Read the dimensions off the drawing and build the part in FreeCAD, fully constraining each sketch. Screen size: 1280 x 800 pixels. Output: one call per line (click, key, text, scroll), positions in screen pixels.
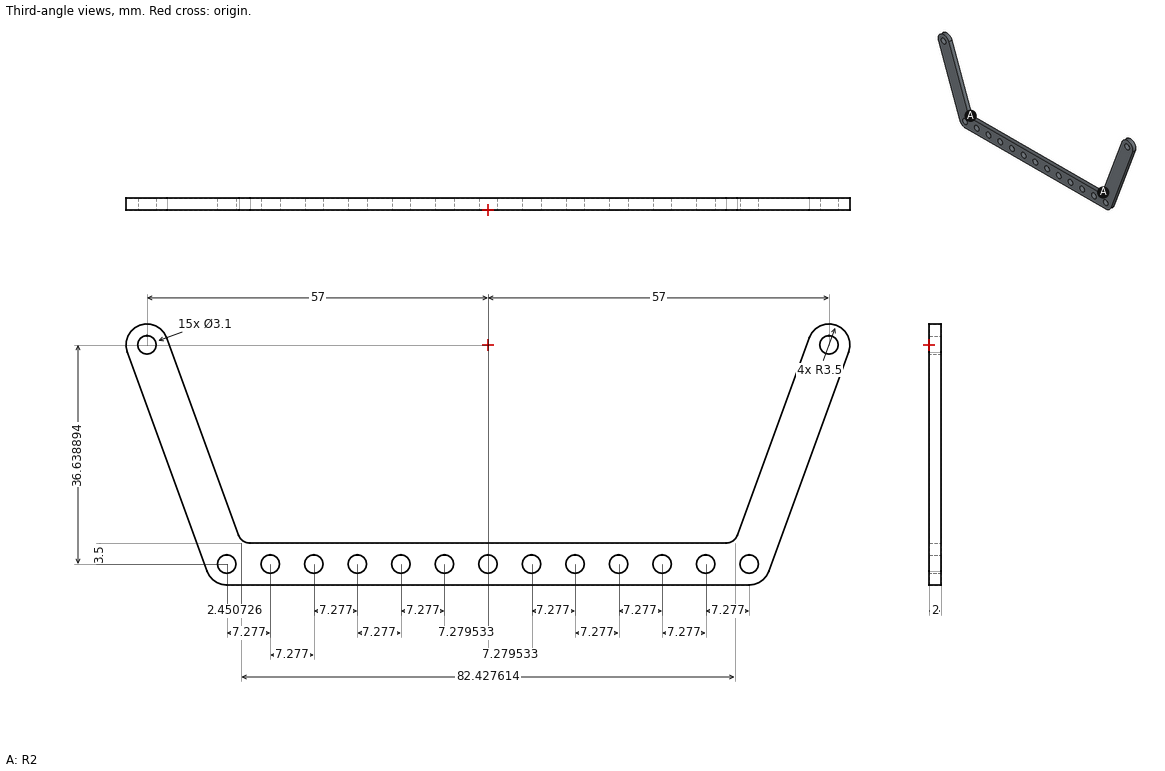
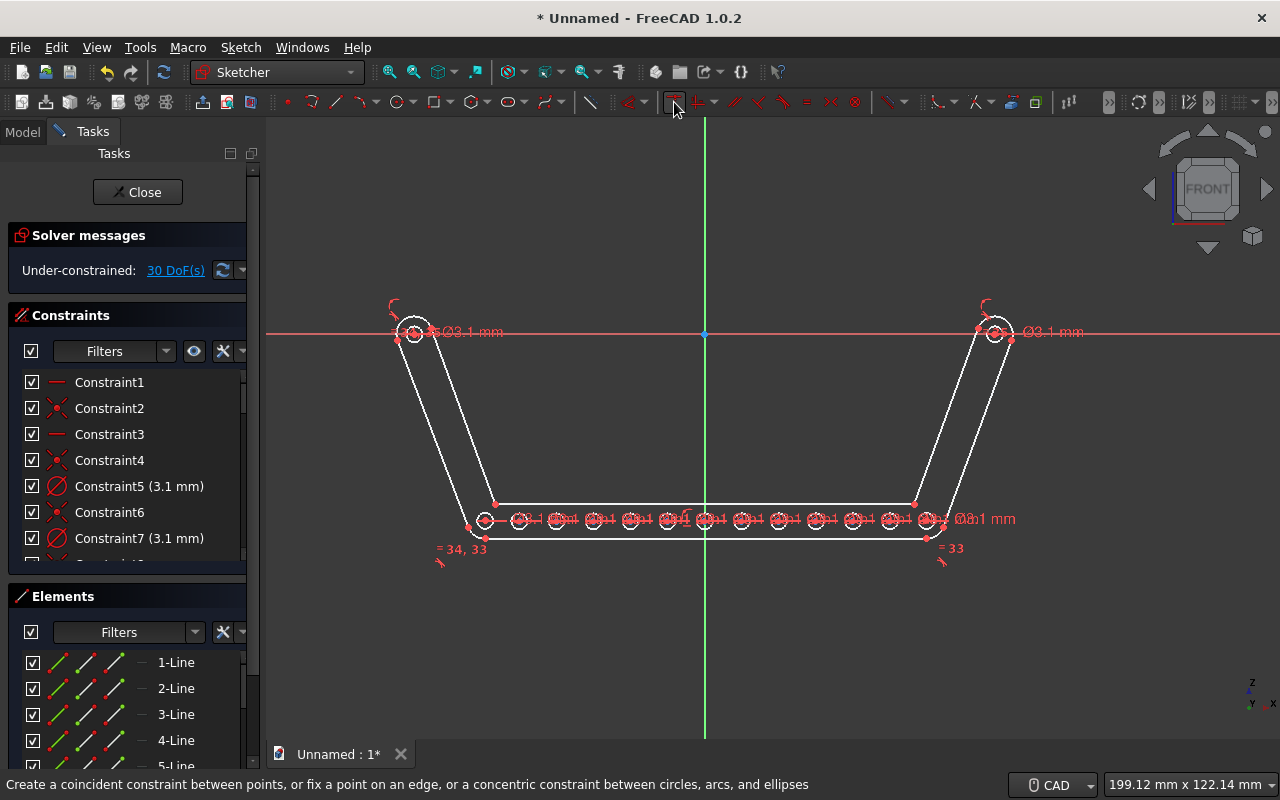
key(d)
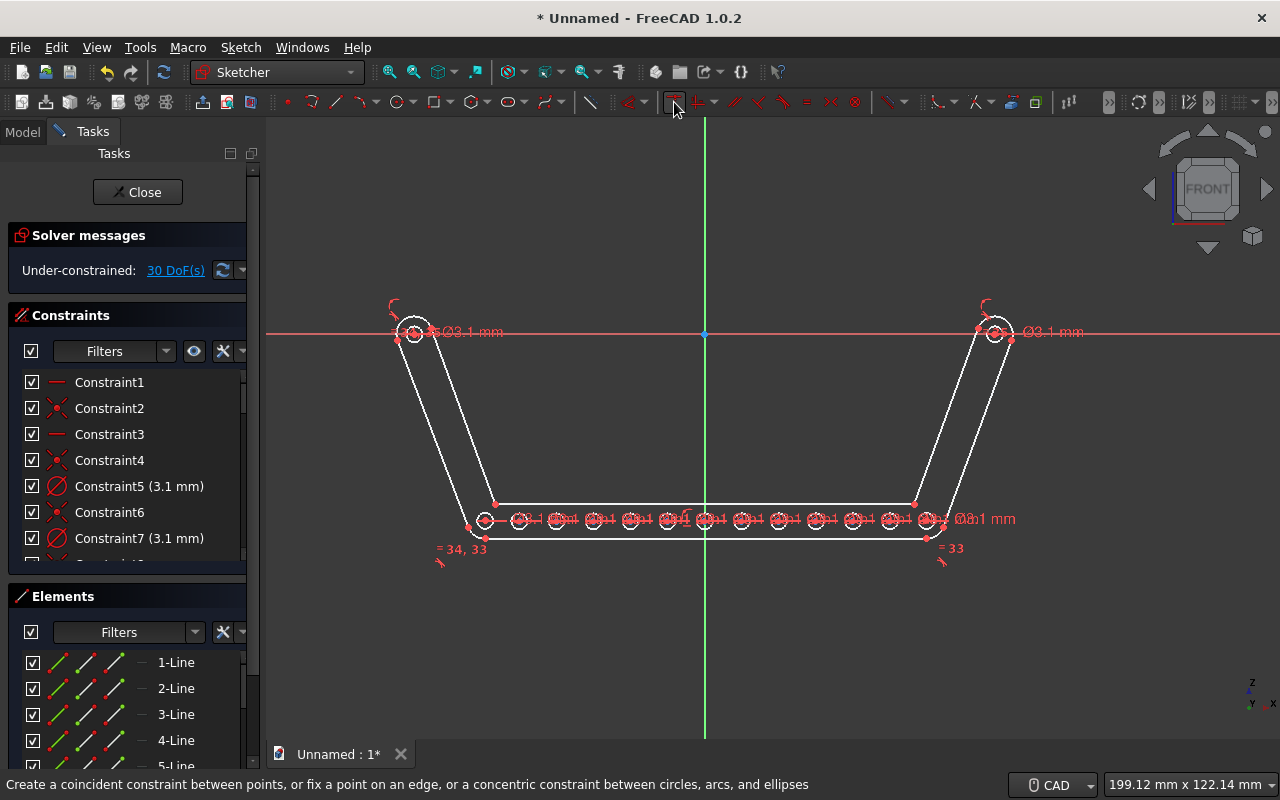
scroll(937, 536, up, 5)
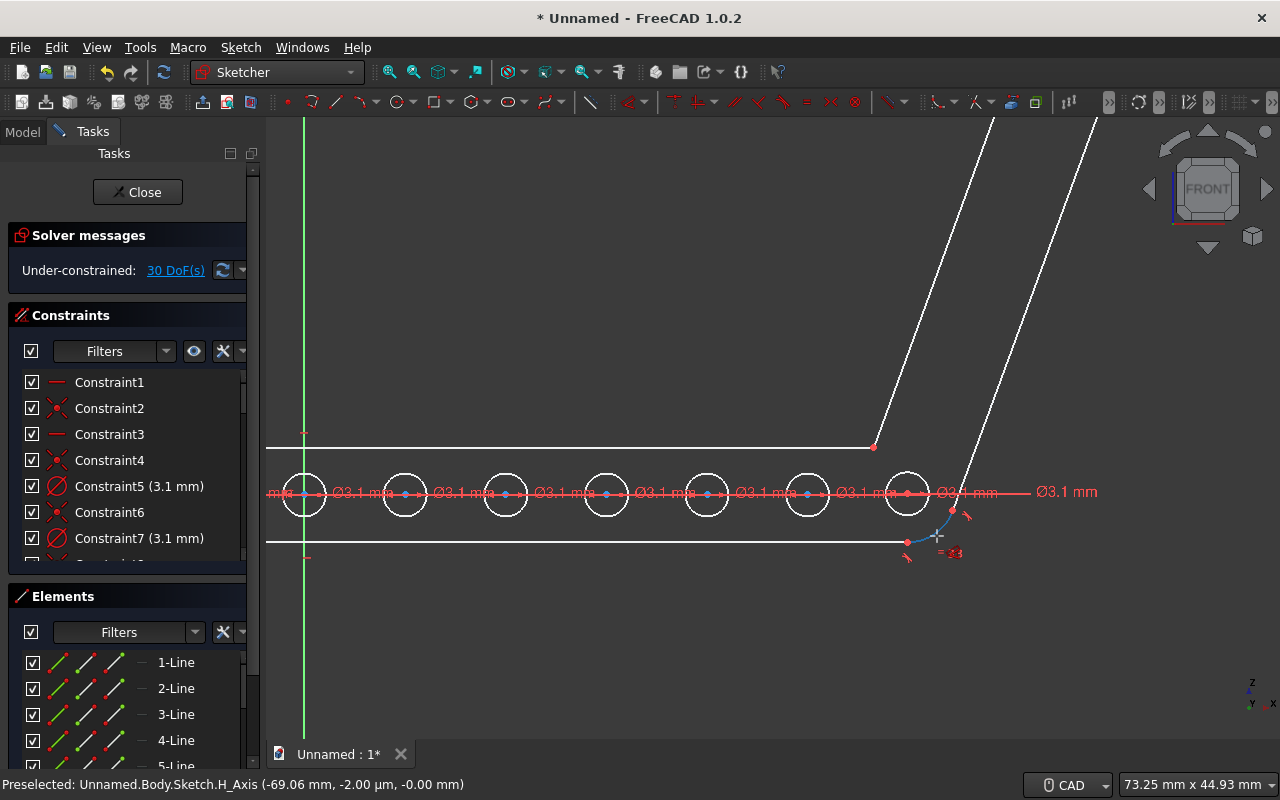
click(935, 534)
click(953, 560)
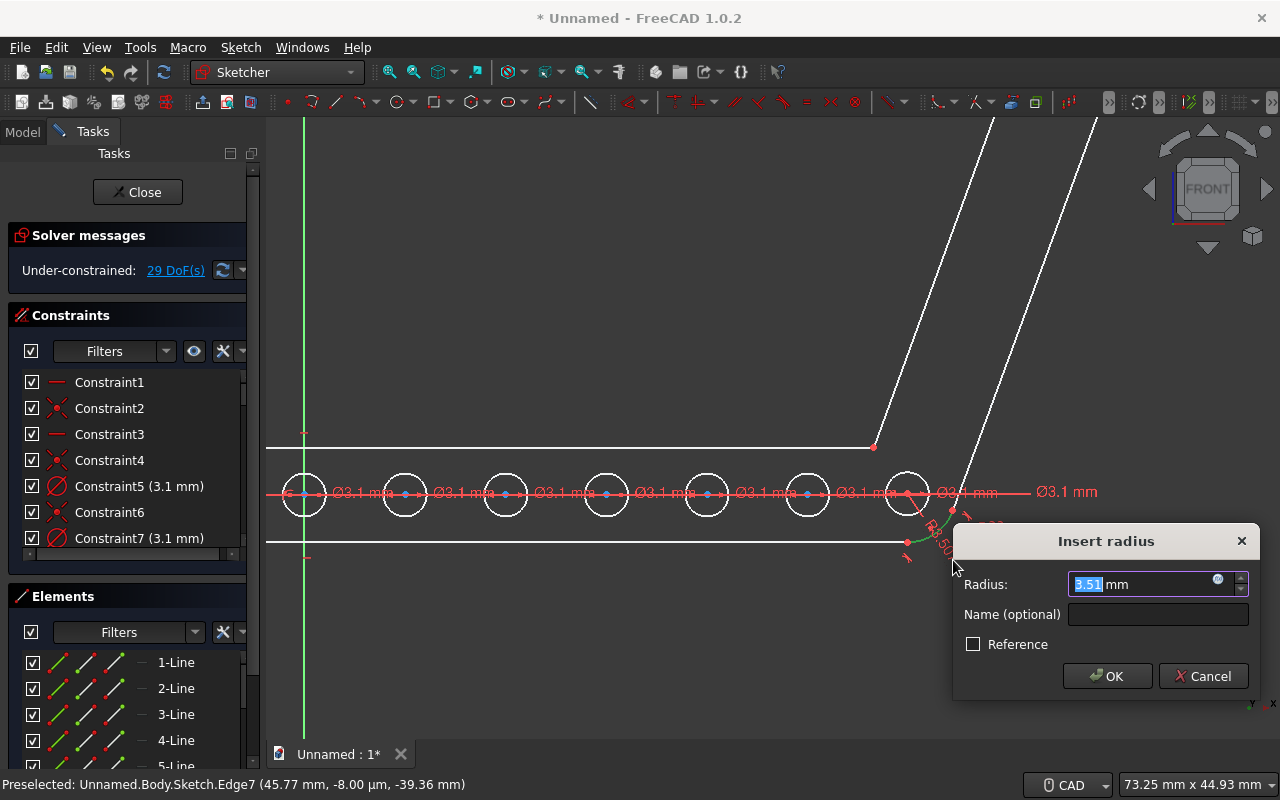
text(3.5)
key(Return)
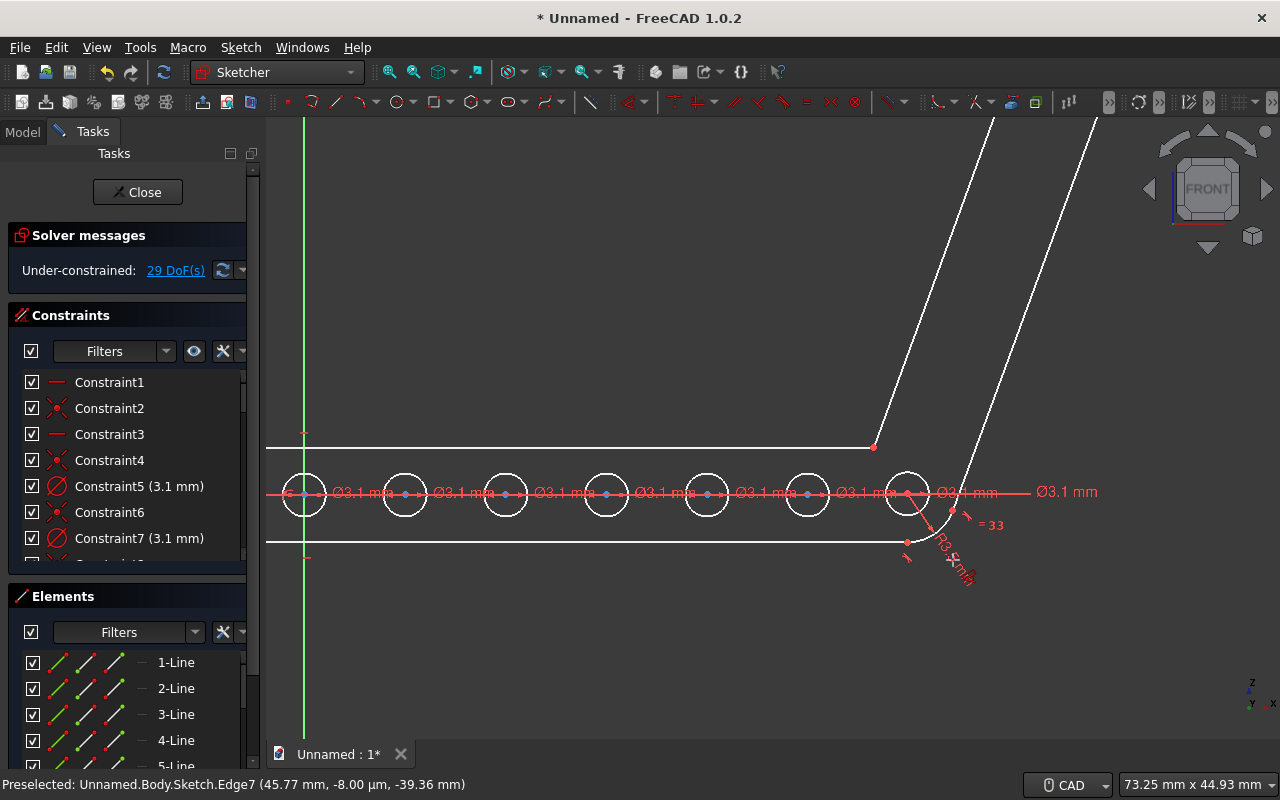
scroll(937, 536, down, 5)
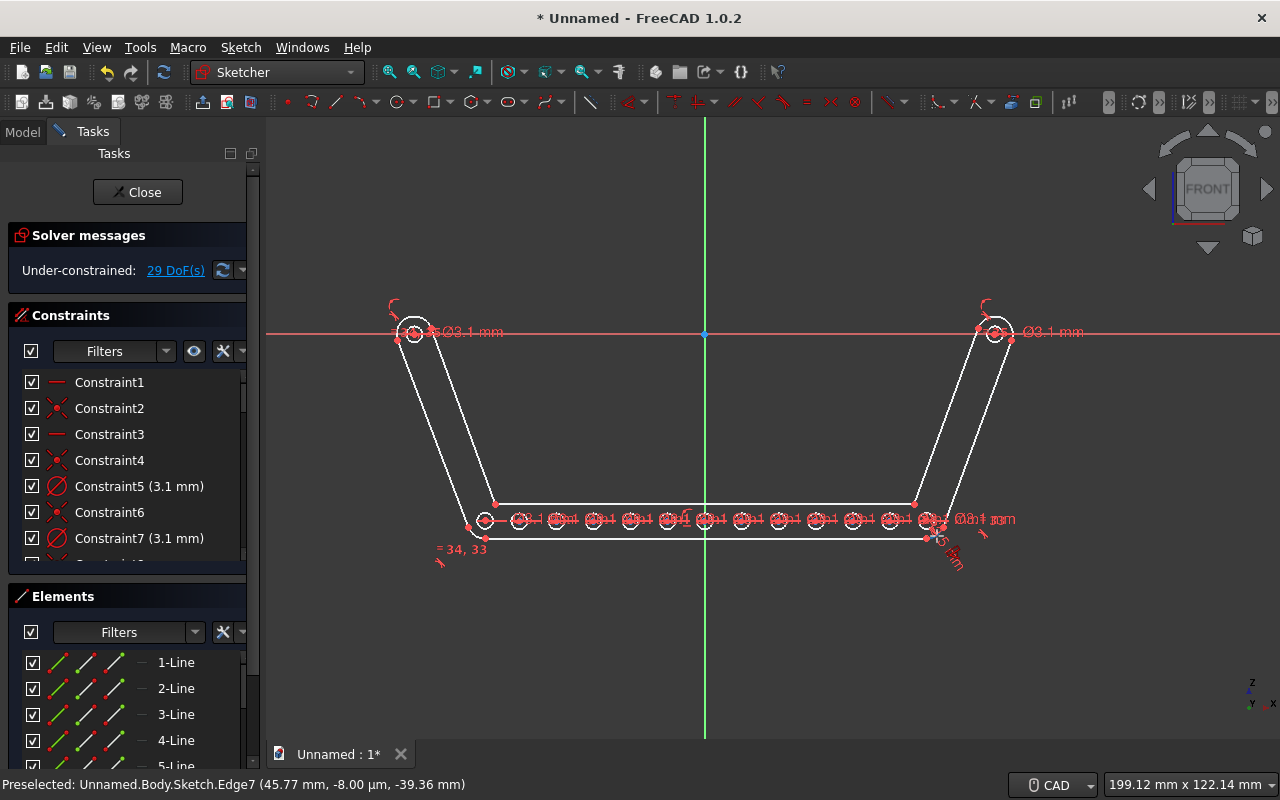
click(414, 334)
click(560, 300)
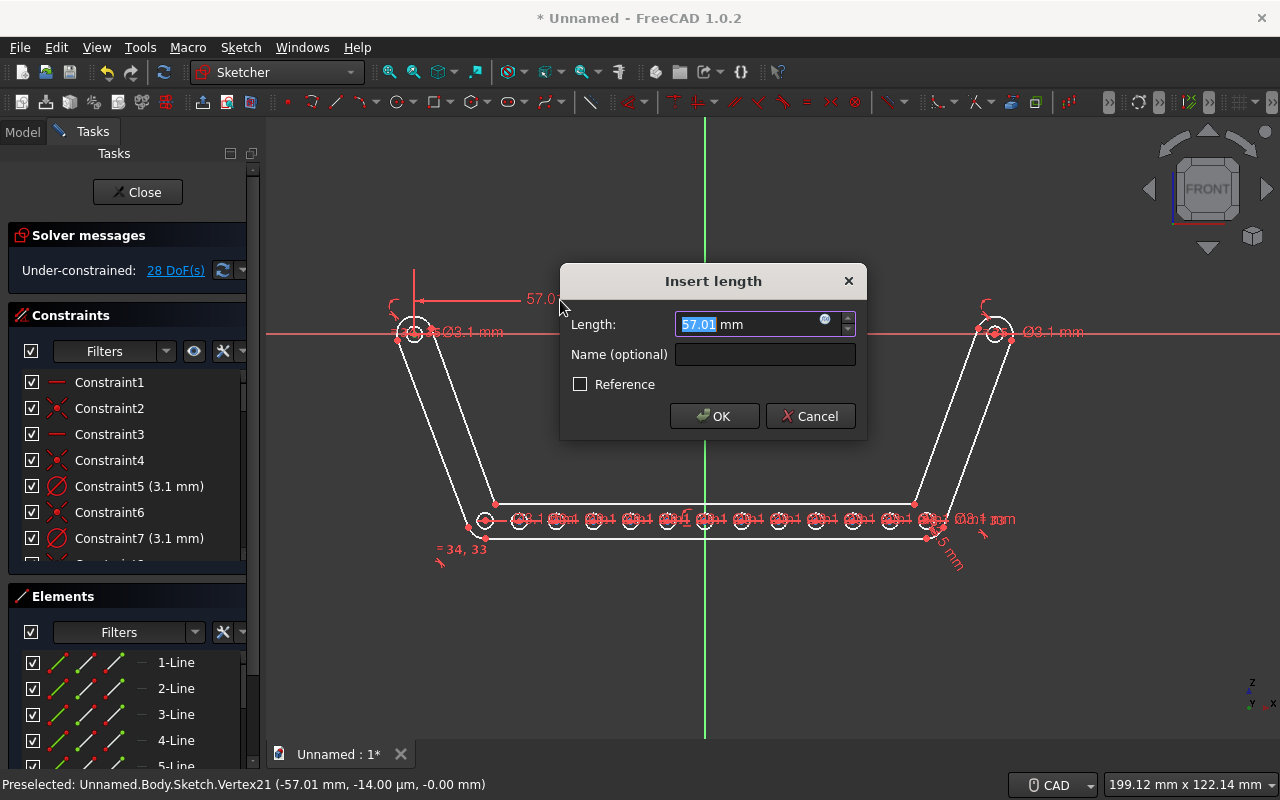
text(57)
key(Return)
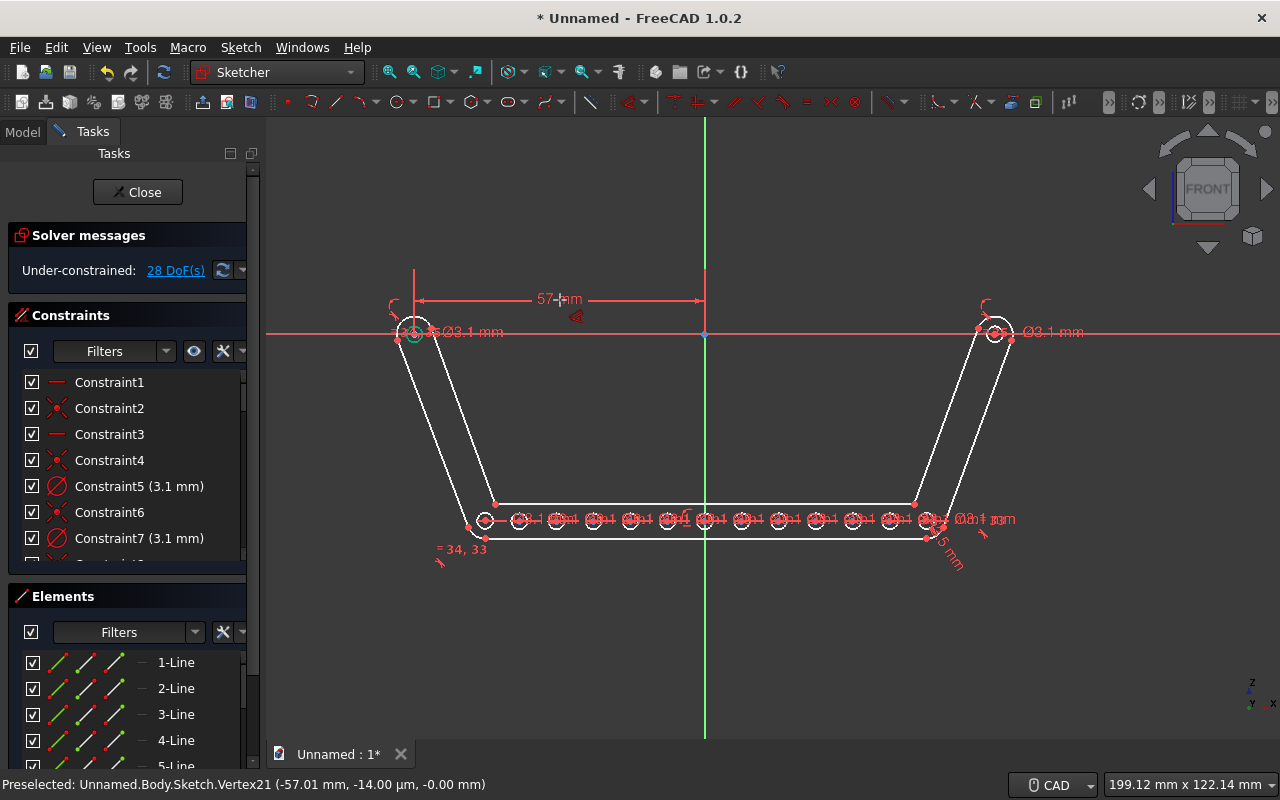
click(995, 334)
click(850, 300)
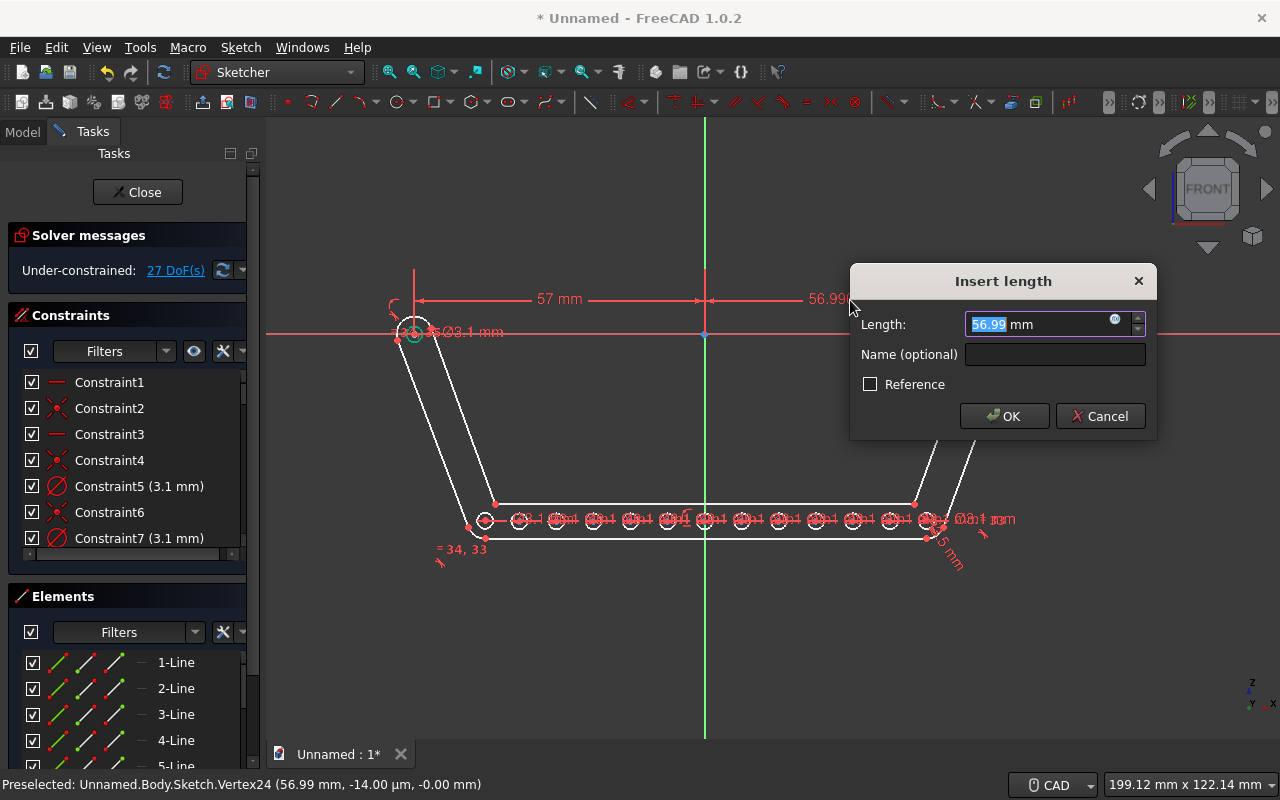
text(57)
key(Return)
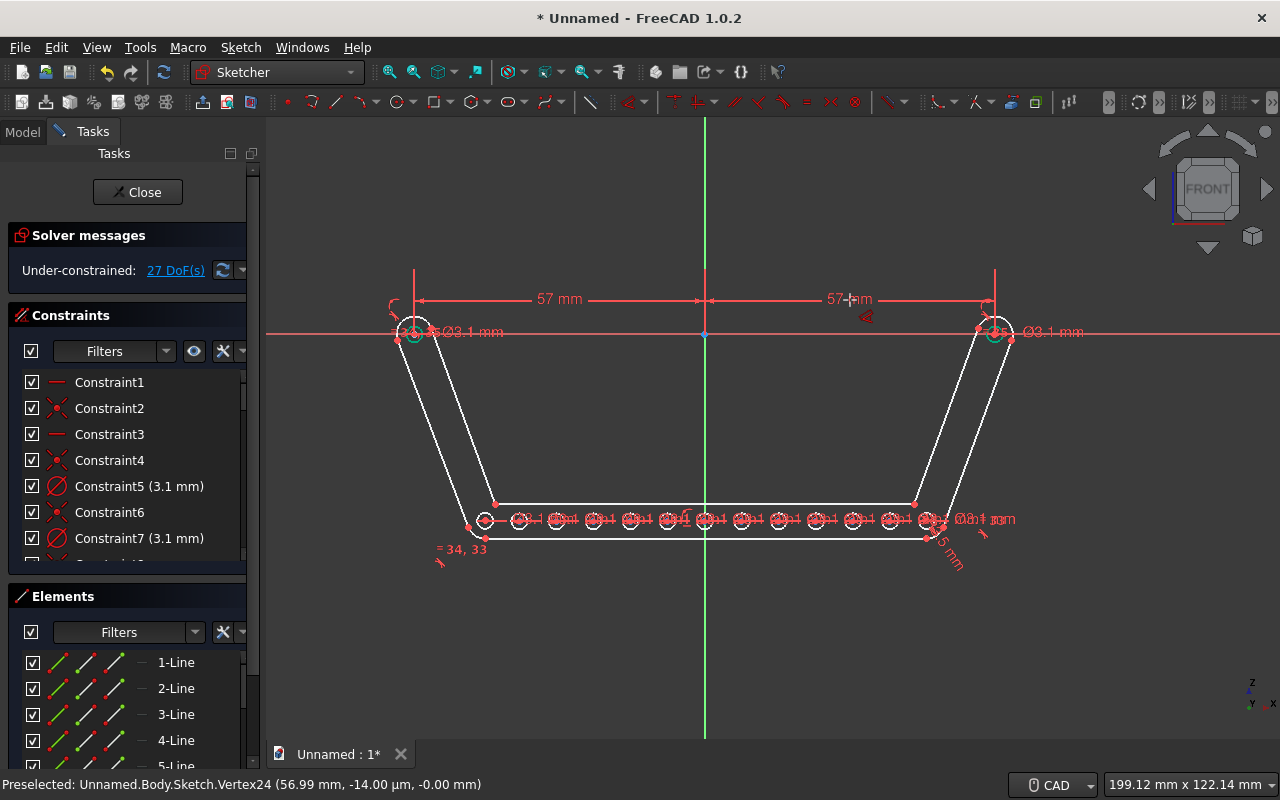
scroll(495, 504, up, 5)